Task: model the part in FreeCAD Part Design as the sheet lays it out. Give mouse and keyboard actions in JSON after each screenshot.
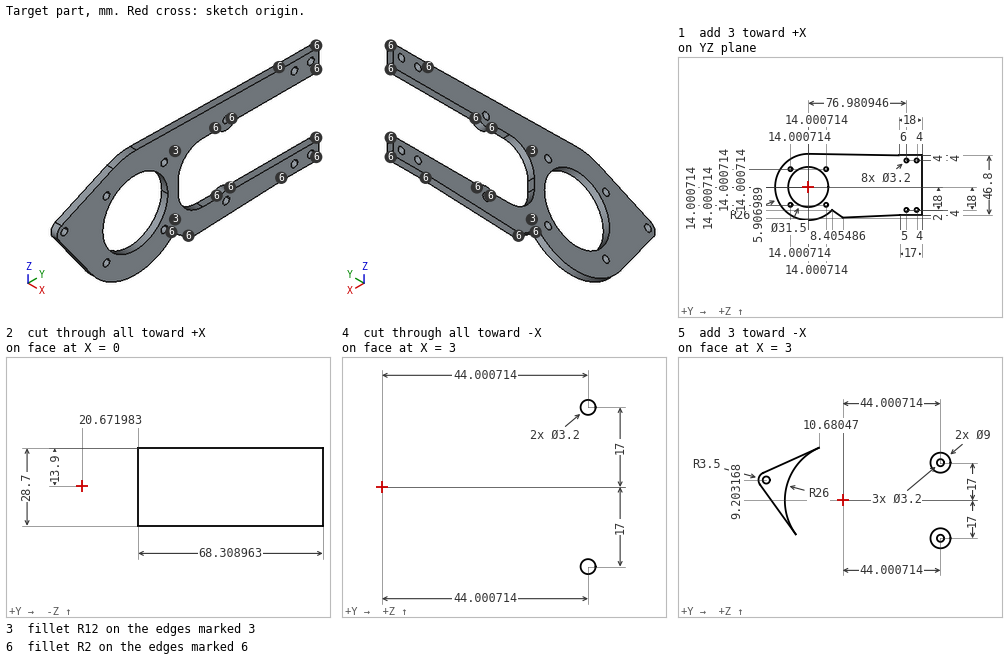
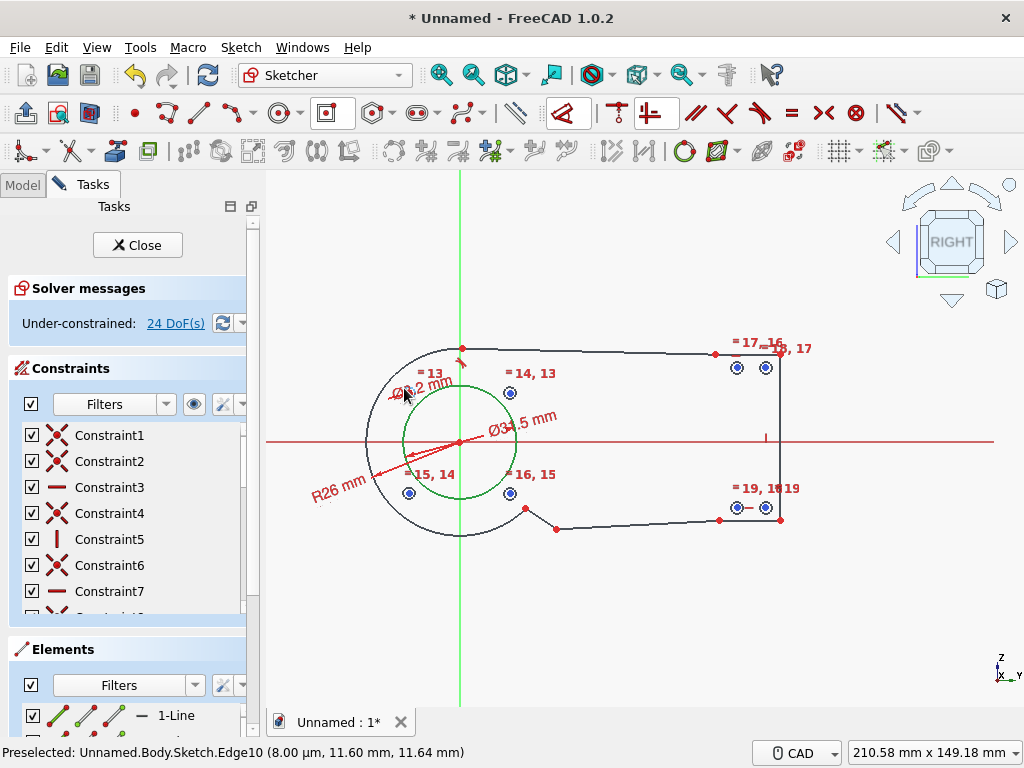
{"action": "scroll", "coordinate": [738, 521], "scroll_direction": "up", "scroll_amount": 4}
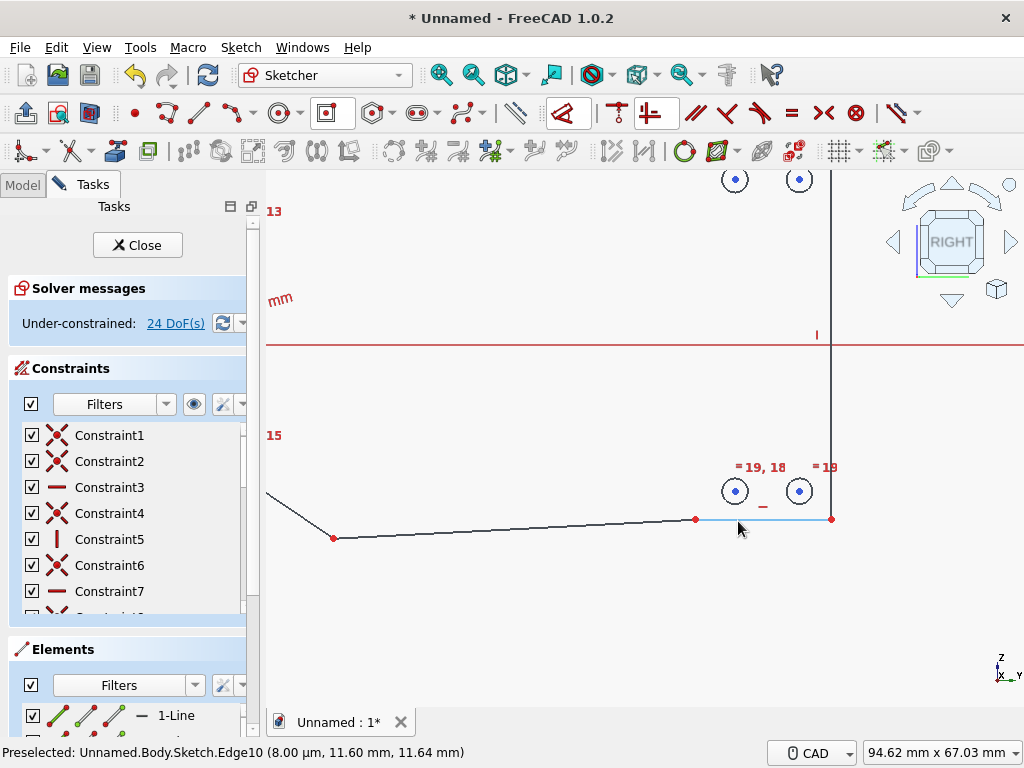
{"action": "left_click", "coordinate": [736, 520]}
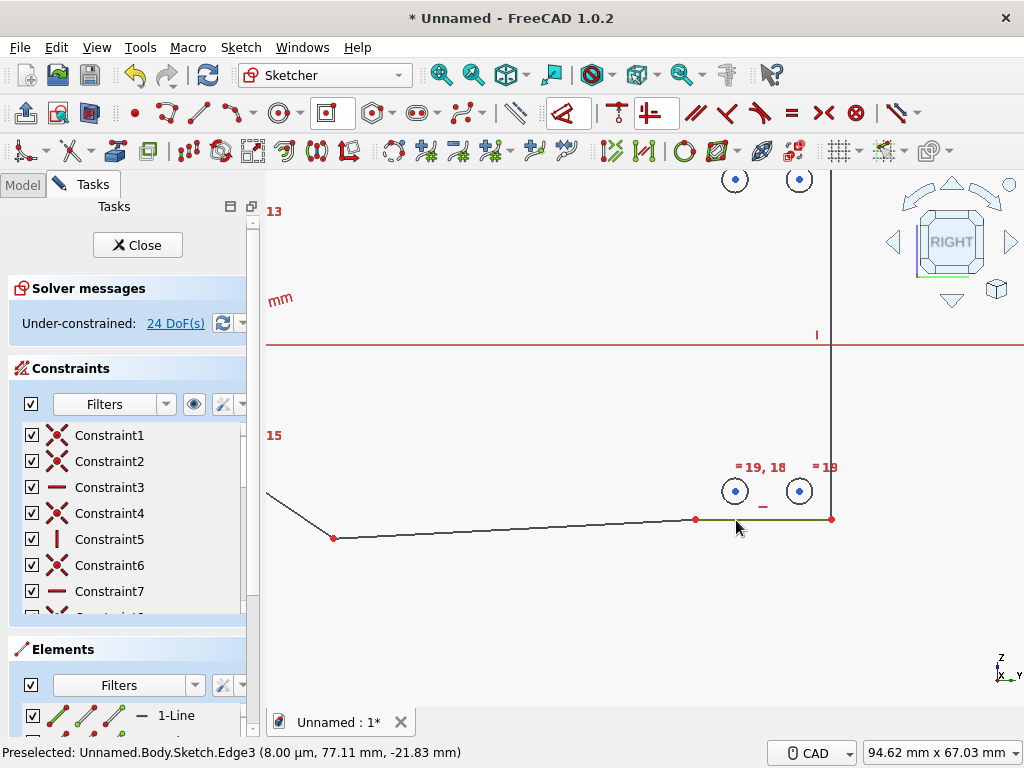
{"action": "left_click", "coordinate": [586, 114]}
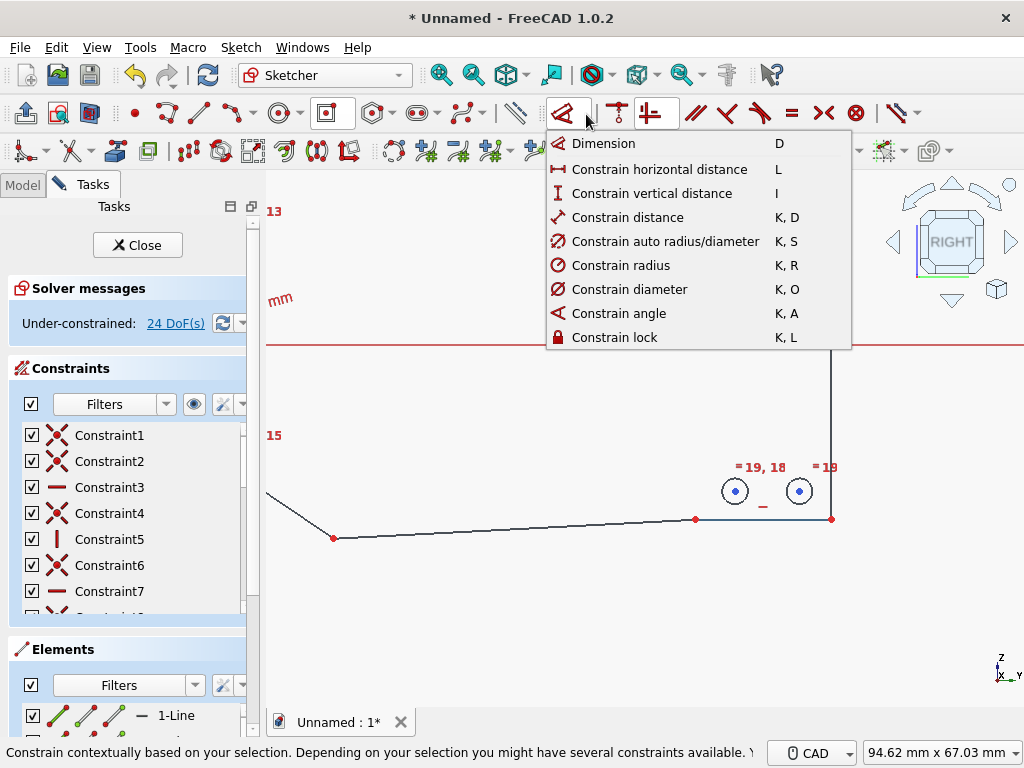
{"action": "left_click", "coordinate": [699, 169]}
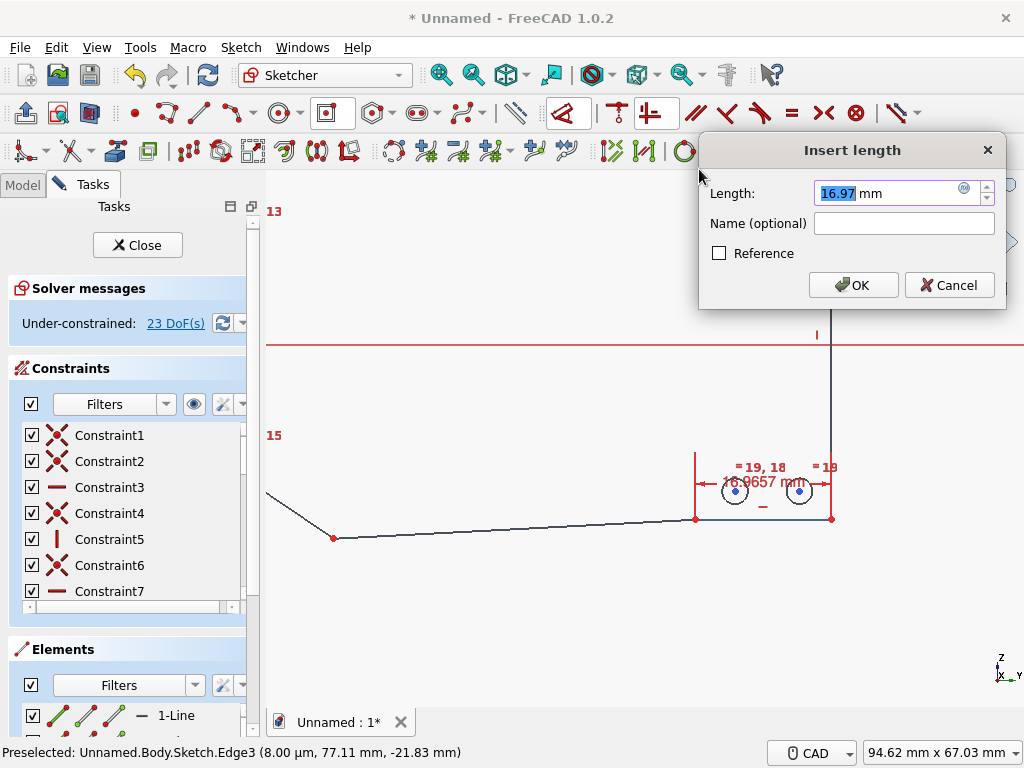
{"action": "type", "text": "17"}
{"action": "key", "text": "Return"}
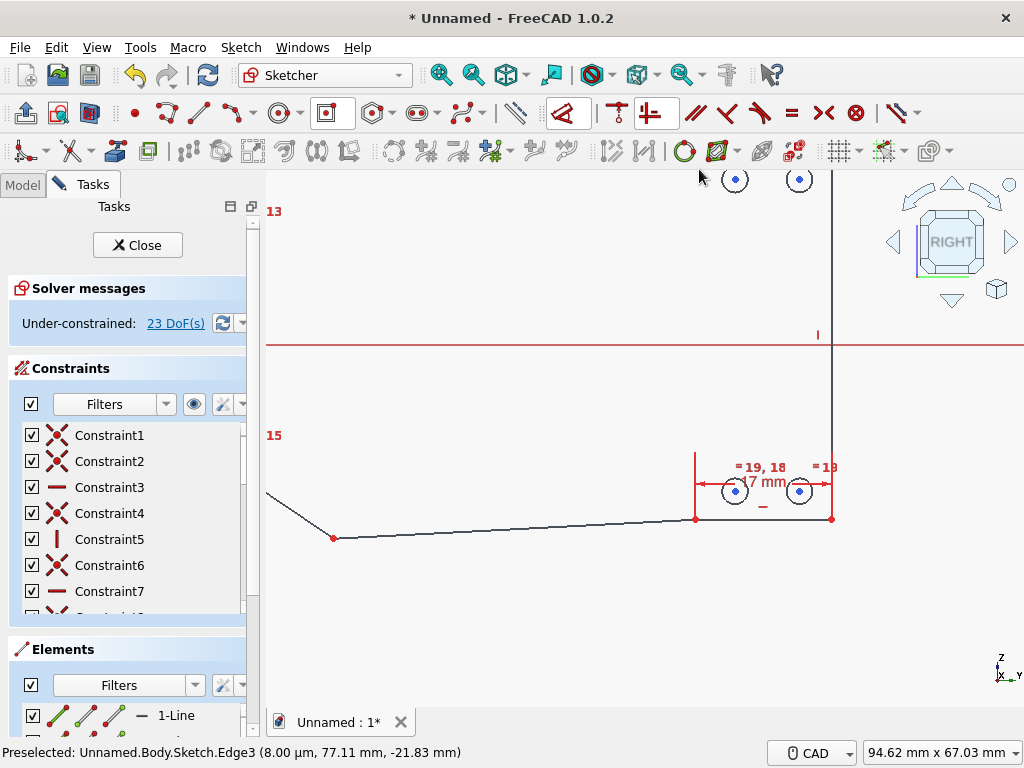
{"action": "scroll", "coordinate": [738, 521], "scroll_direction": "down", "scroll_amount": 4}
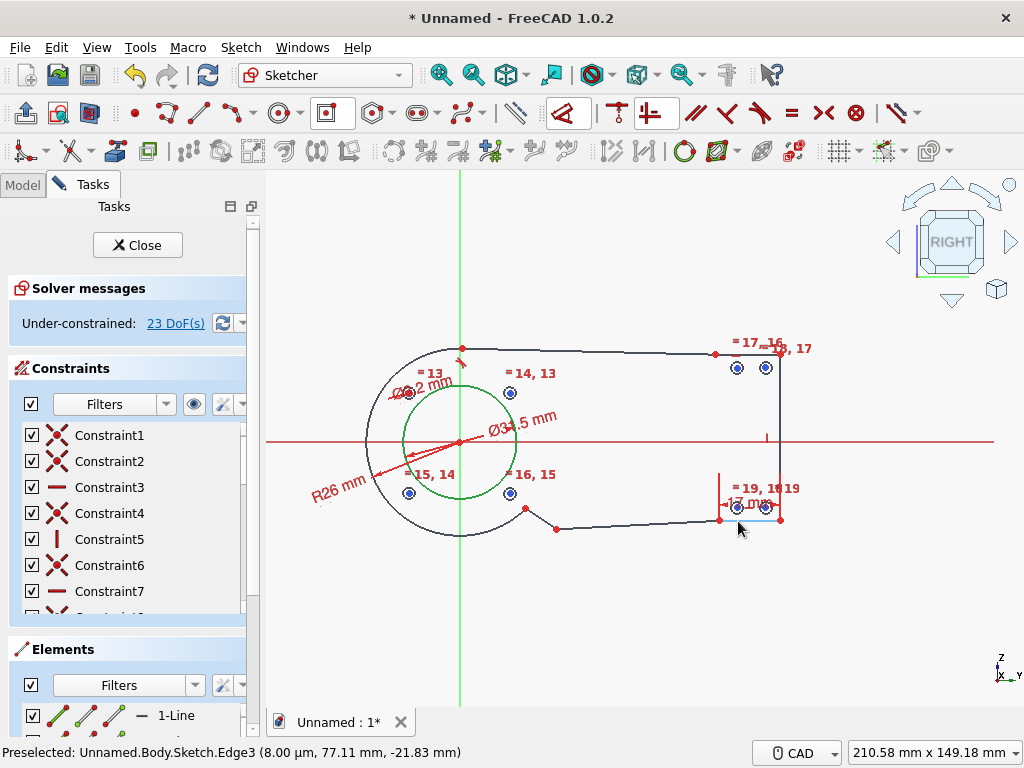
{"action": "scroll", "coordinate": [761, 355], "scroll_direction": "up", "scroll_amount": 3}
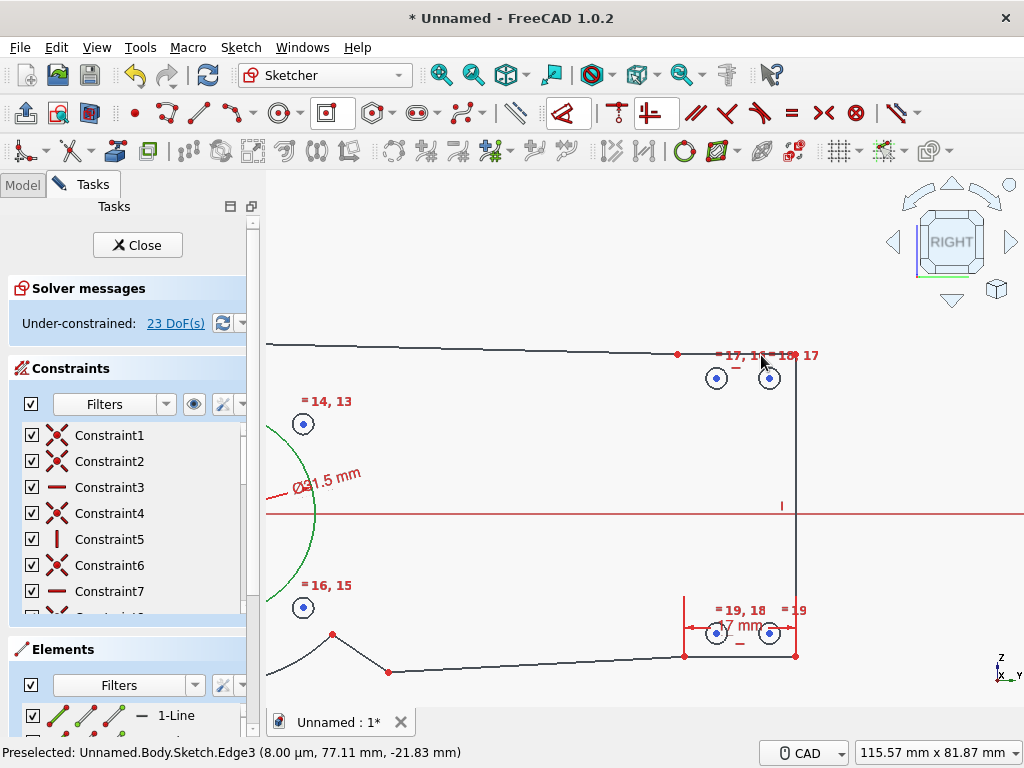
{"action": "left_click", "coordinate": [713, 354]}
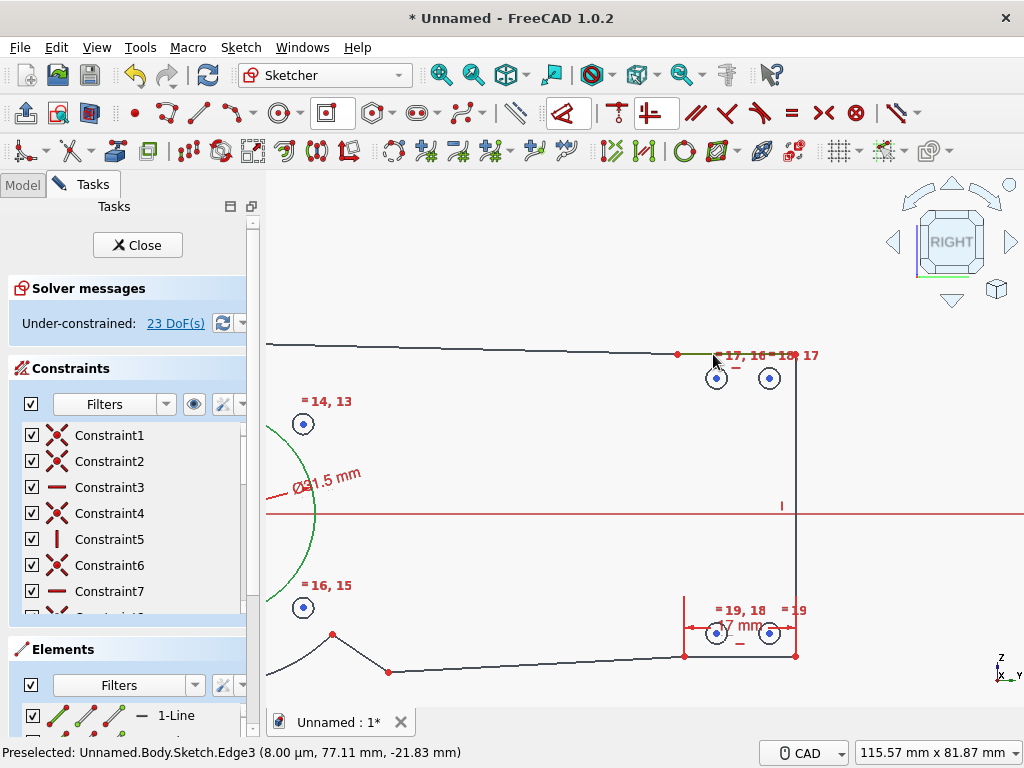
{"action": "key", "text": "l"}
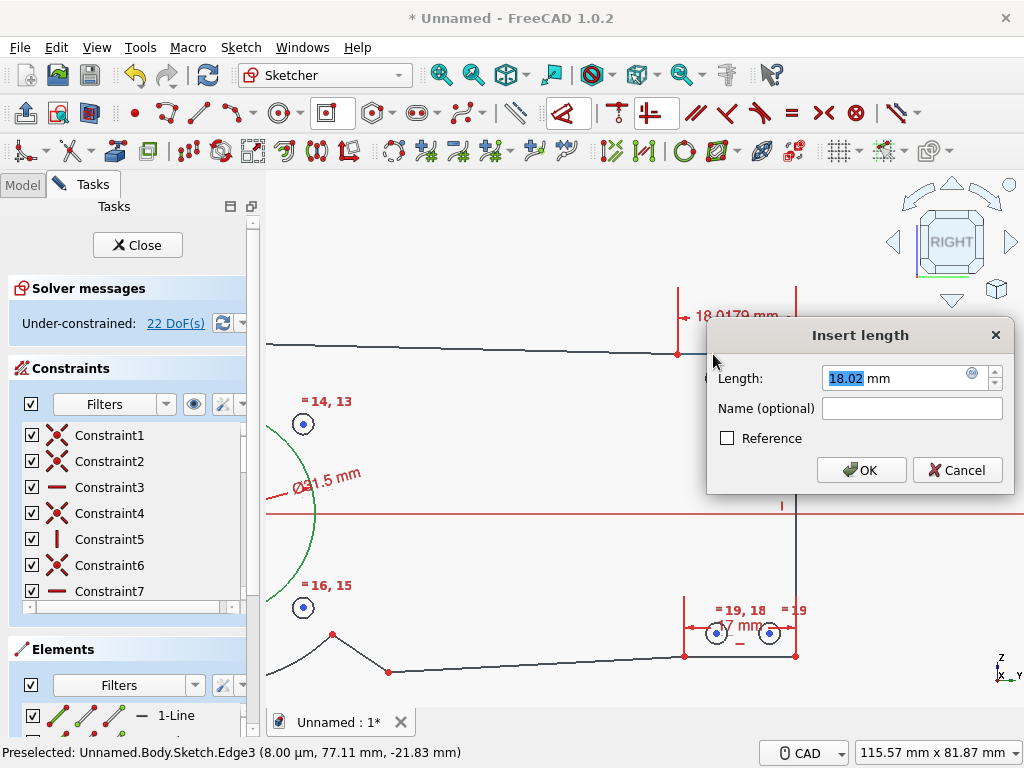
{"action": "type", "text": "18"}
{"action": "key", "text": "Return"}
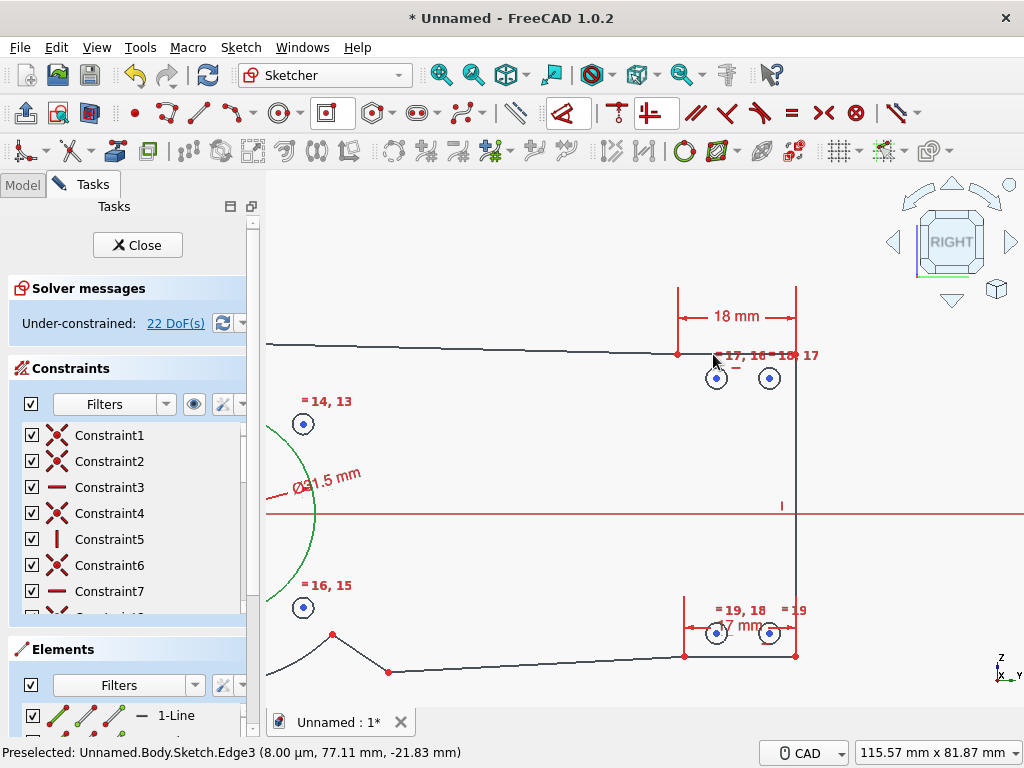
{"action": "scroll", "coordinate": [477, 668], "scroll_direction": "up", "scroll_amount": 6}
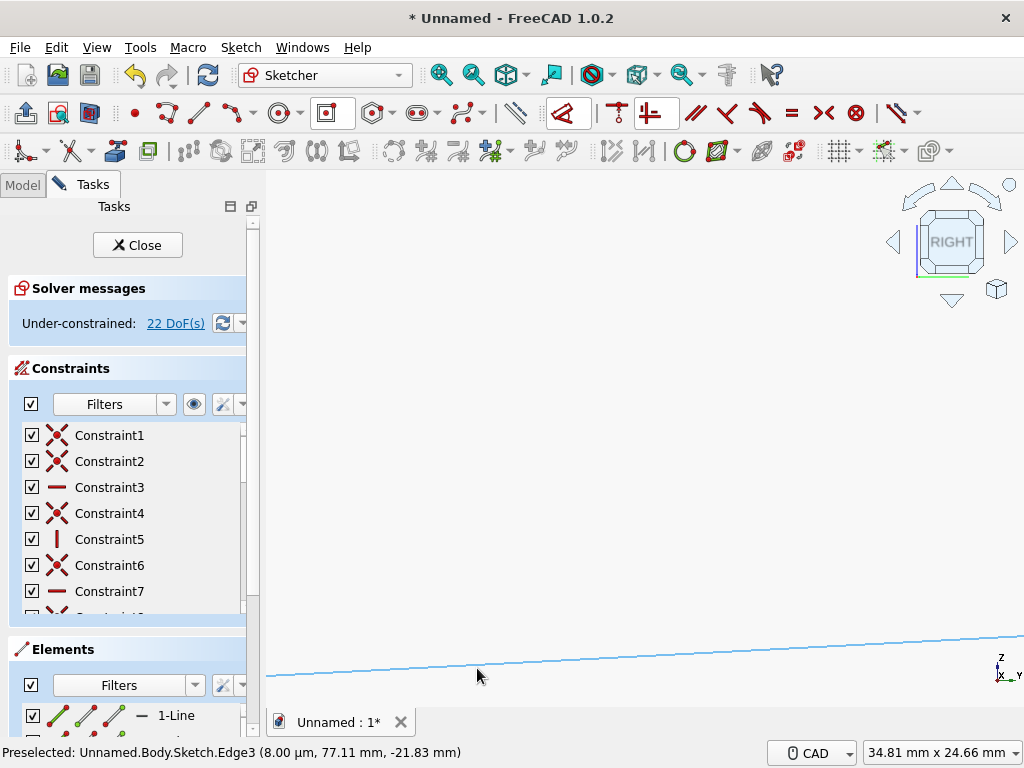
{"action": "left_click", "coordinate": [477, 665]}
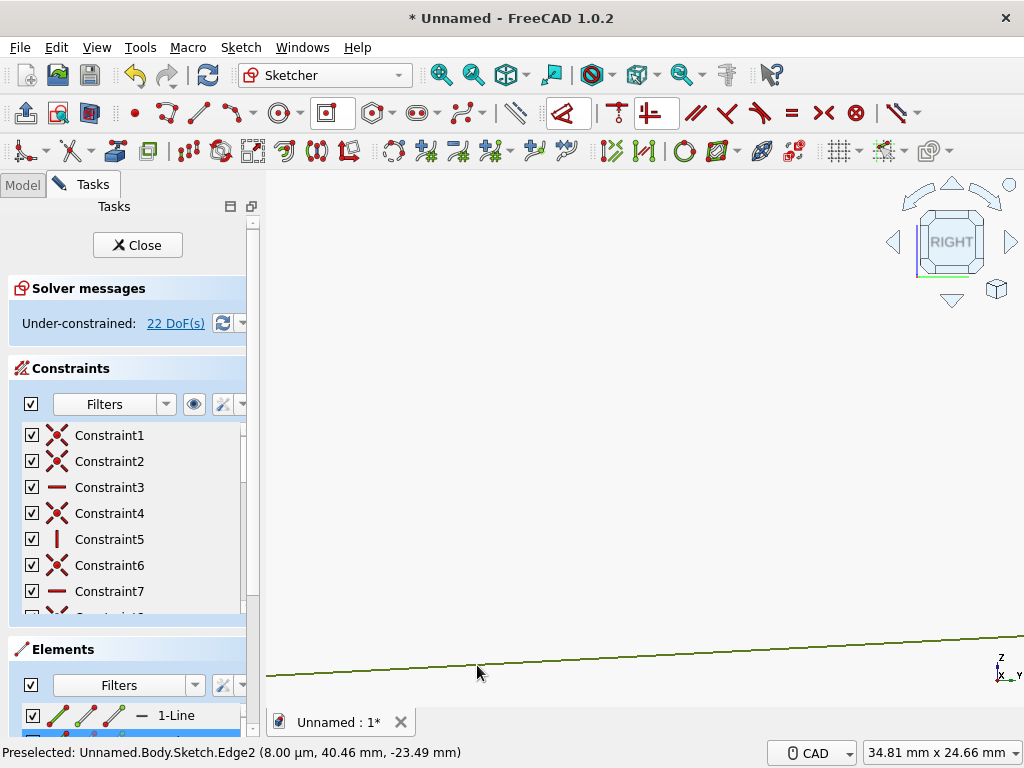
{"action": "key", "text": "i"}